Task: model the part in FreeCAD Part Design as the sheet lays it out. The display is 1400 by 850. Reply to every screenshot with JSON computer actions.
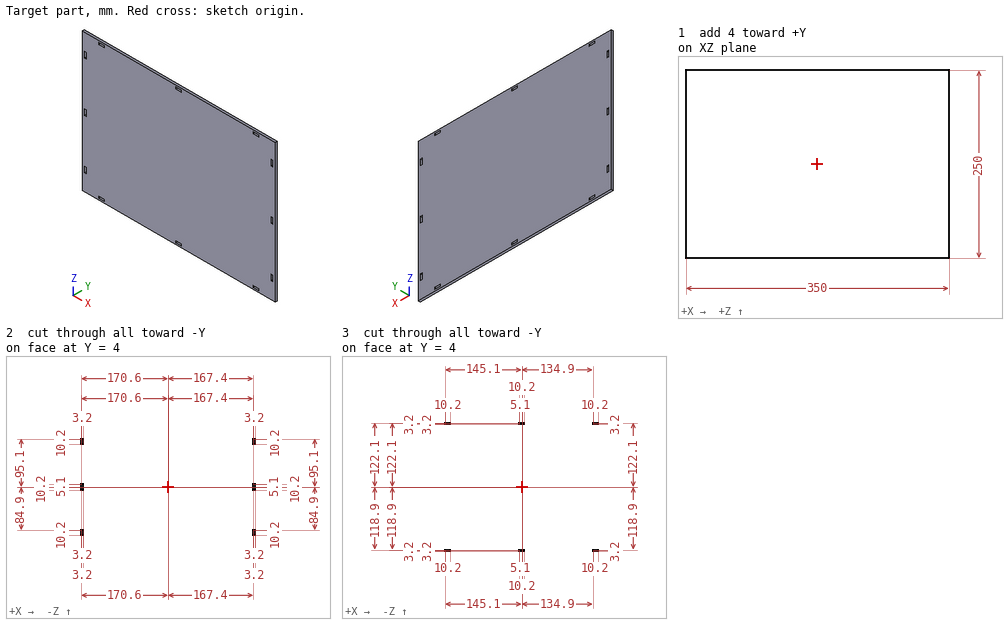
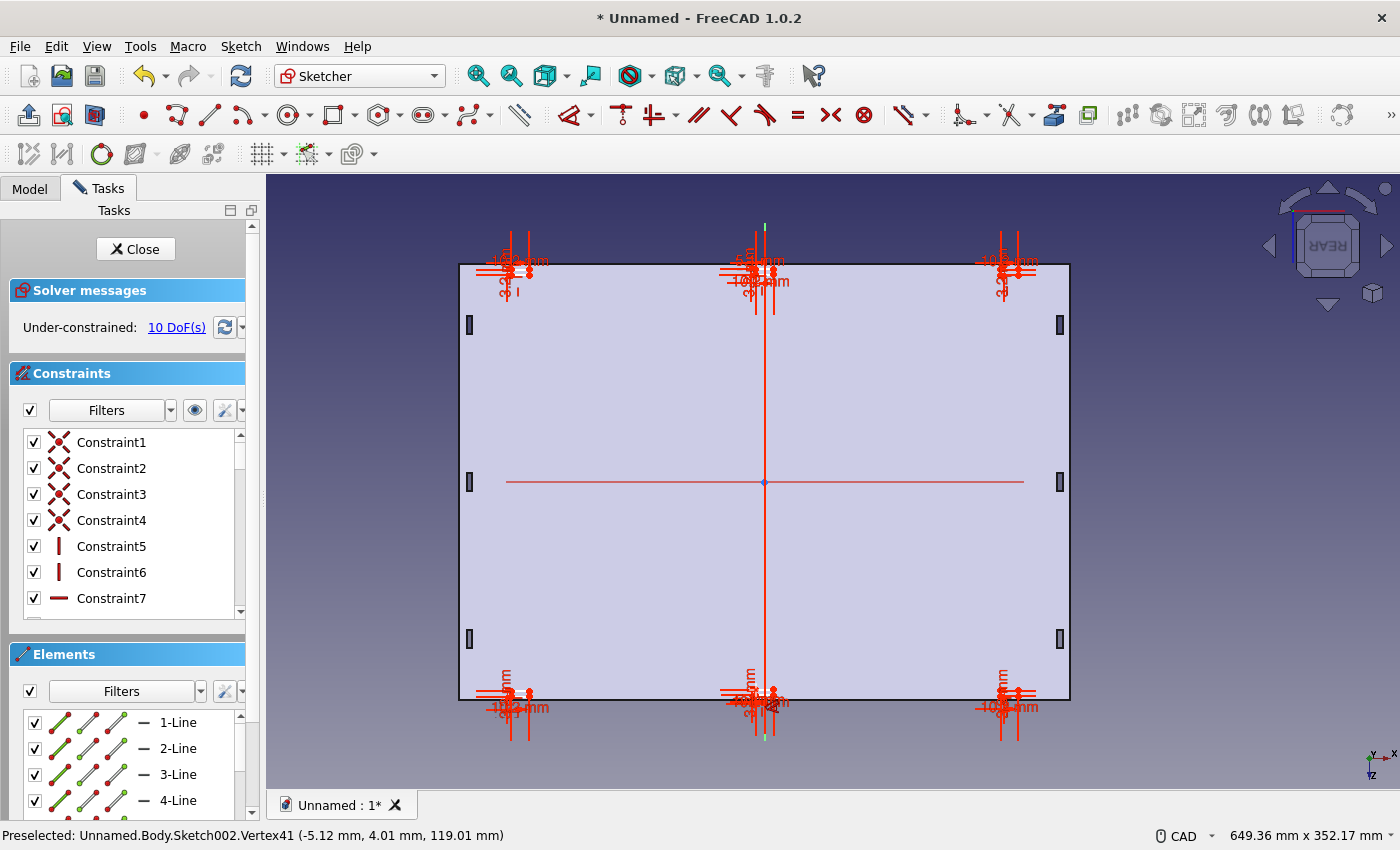
{"action": "scroll", "coordinate": [756, 269], "scroll_direction": "up", "scroll_amount": 4}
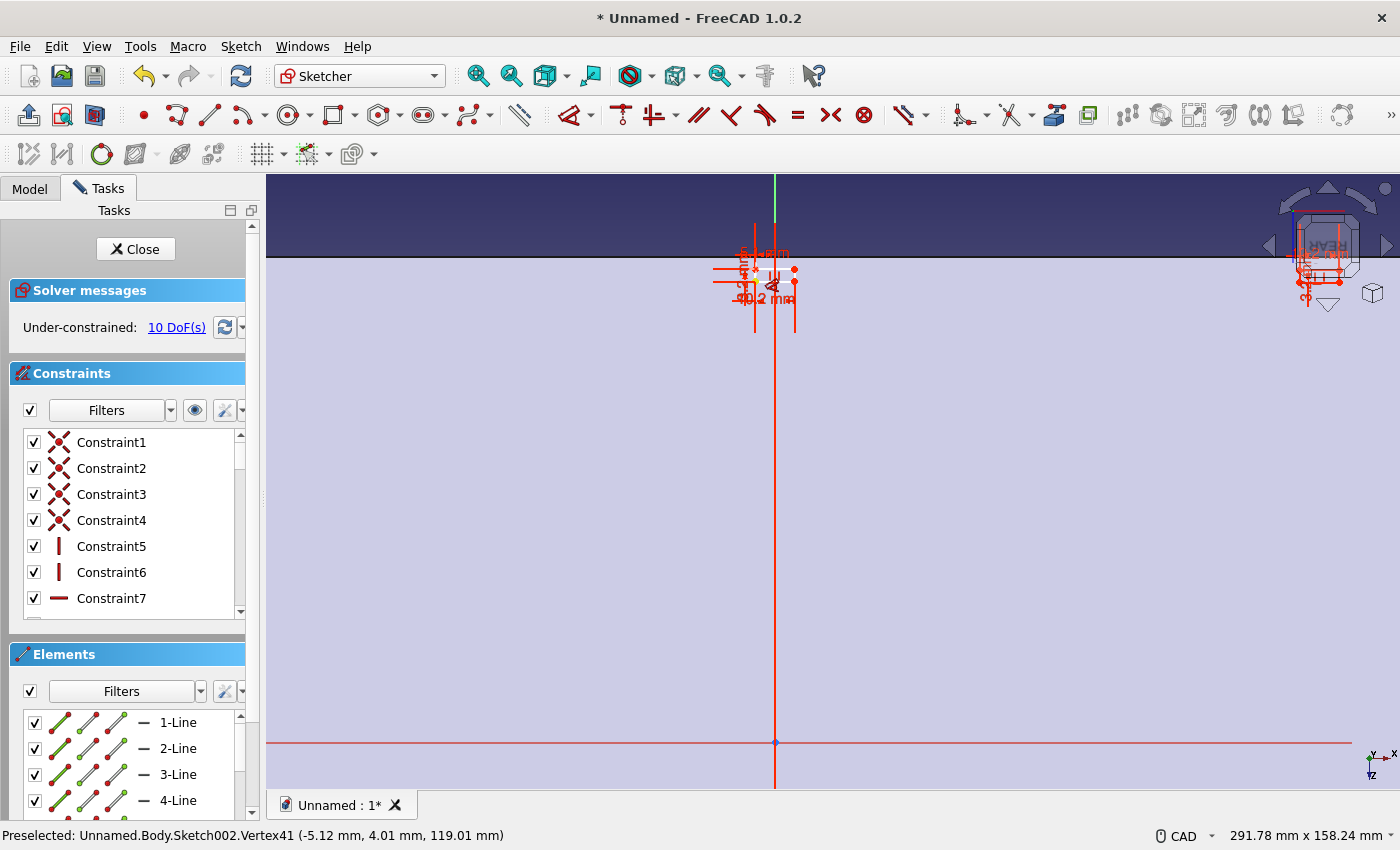
{"action": "left_click", "coordinate": [755, 269]}
{"action": "left_click", "coordinate": [721, 506]}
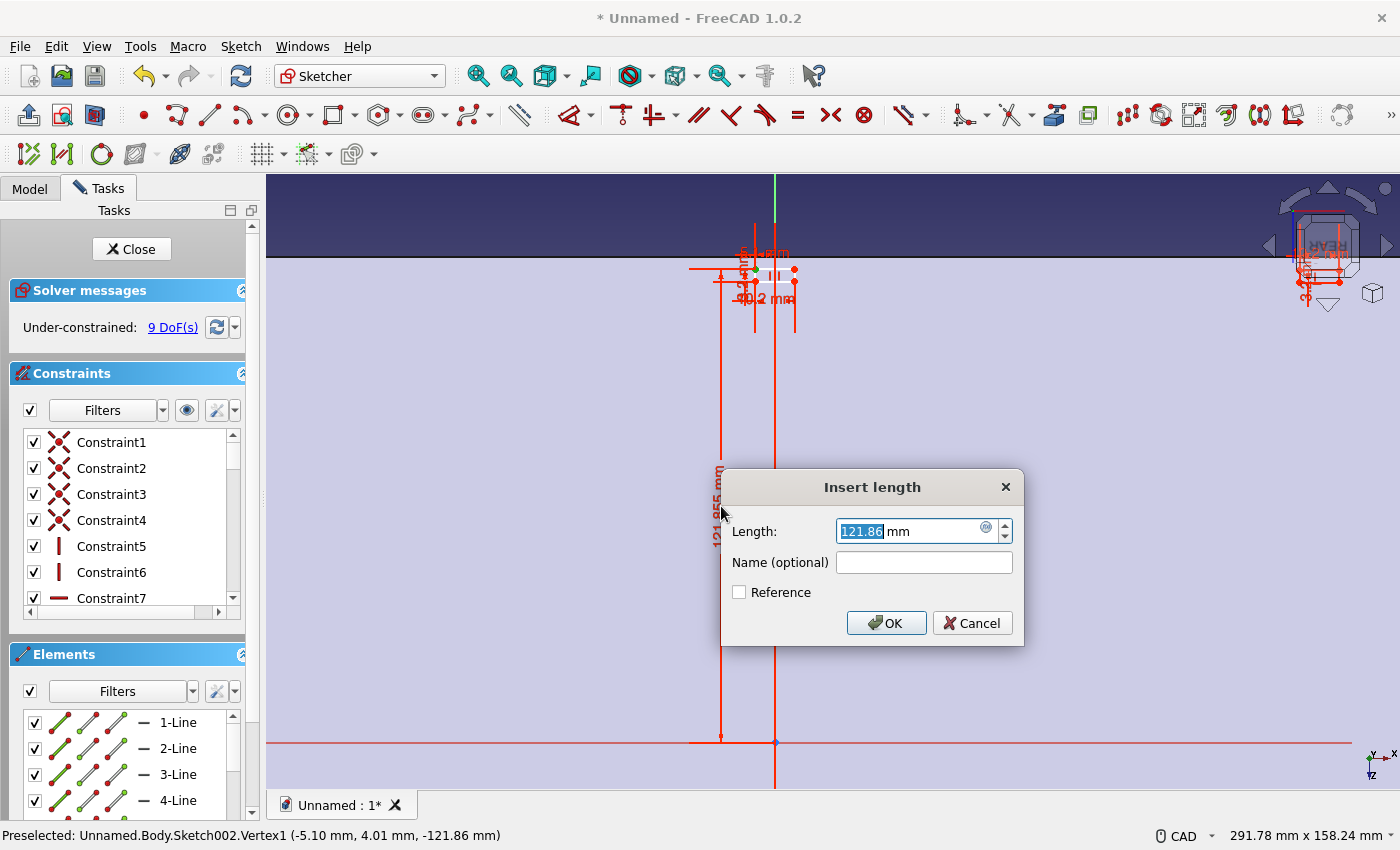
{"action": "type", "text": "122.1"}
{"action": "key", "text": "Return"}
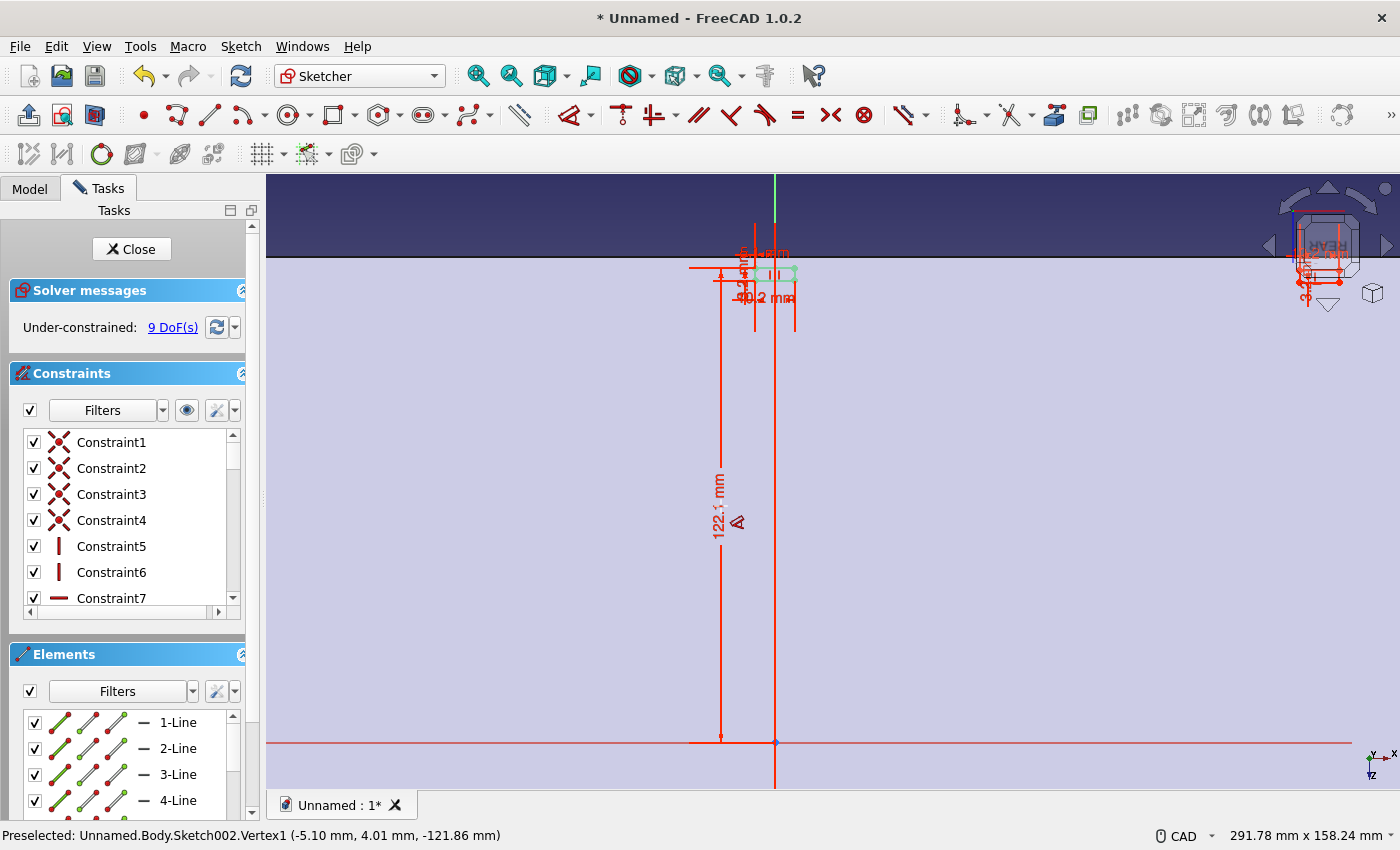
{"action": "scroll", "coordinate": [756, 268], "scroll_direction": "down", "scroll_amount": 4}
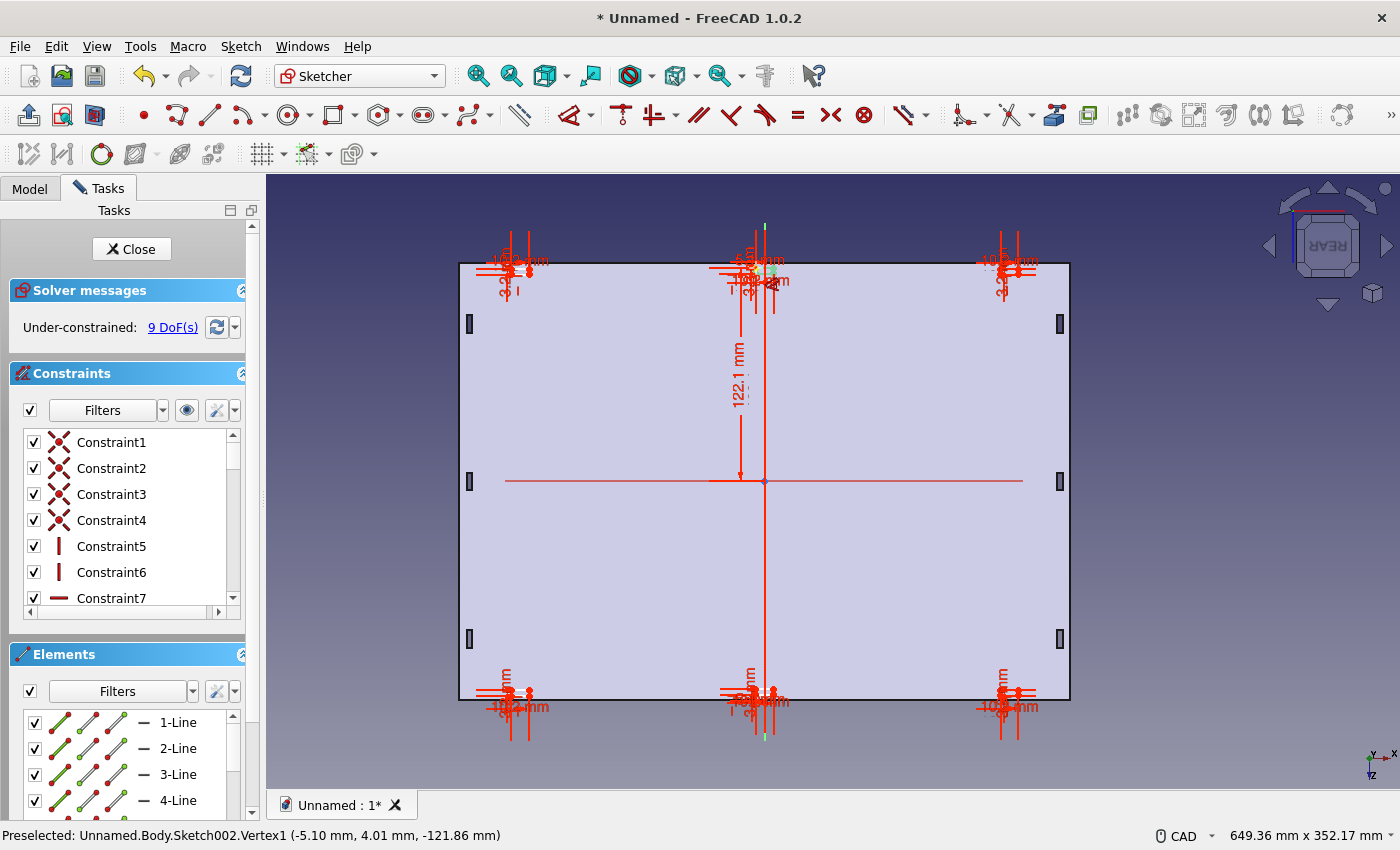
{"action": "scroll", "coordinate": [1001, 269], "scroll_direction": "up", "scroll_amount": 4}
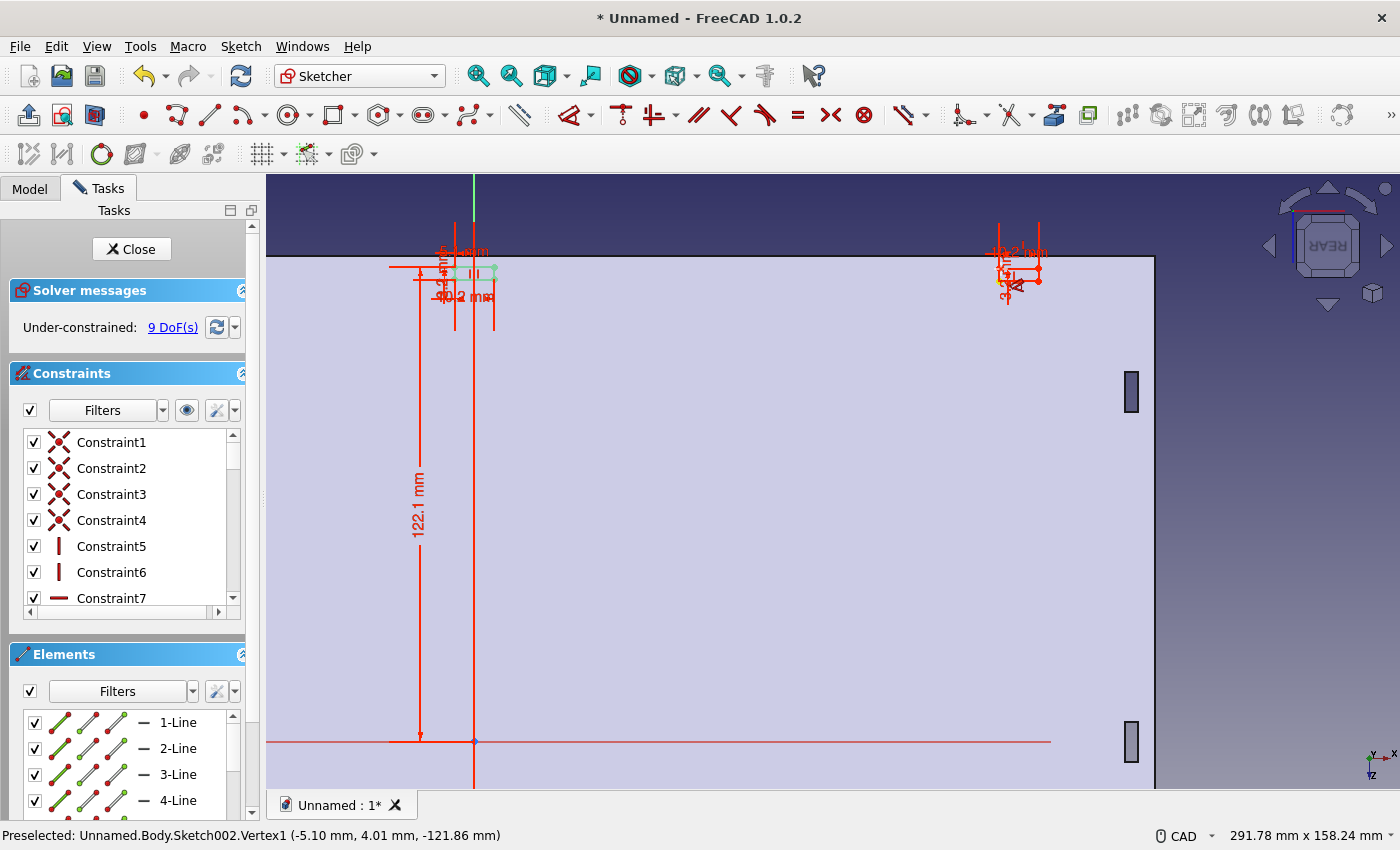
{"action": "left_click", "coordinate": [999, 269]}
{"action": "left_click", "coordinate": [737, 235]}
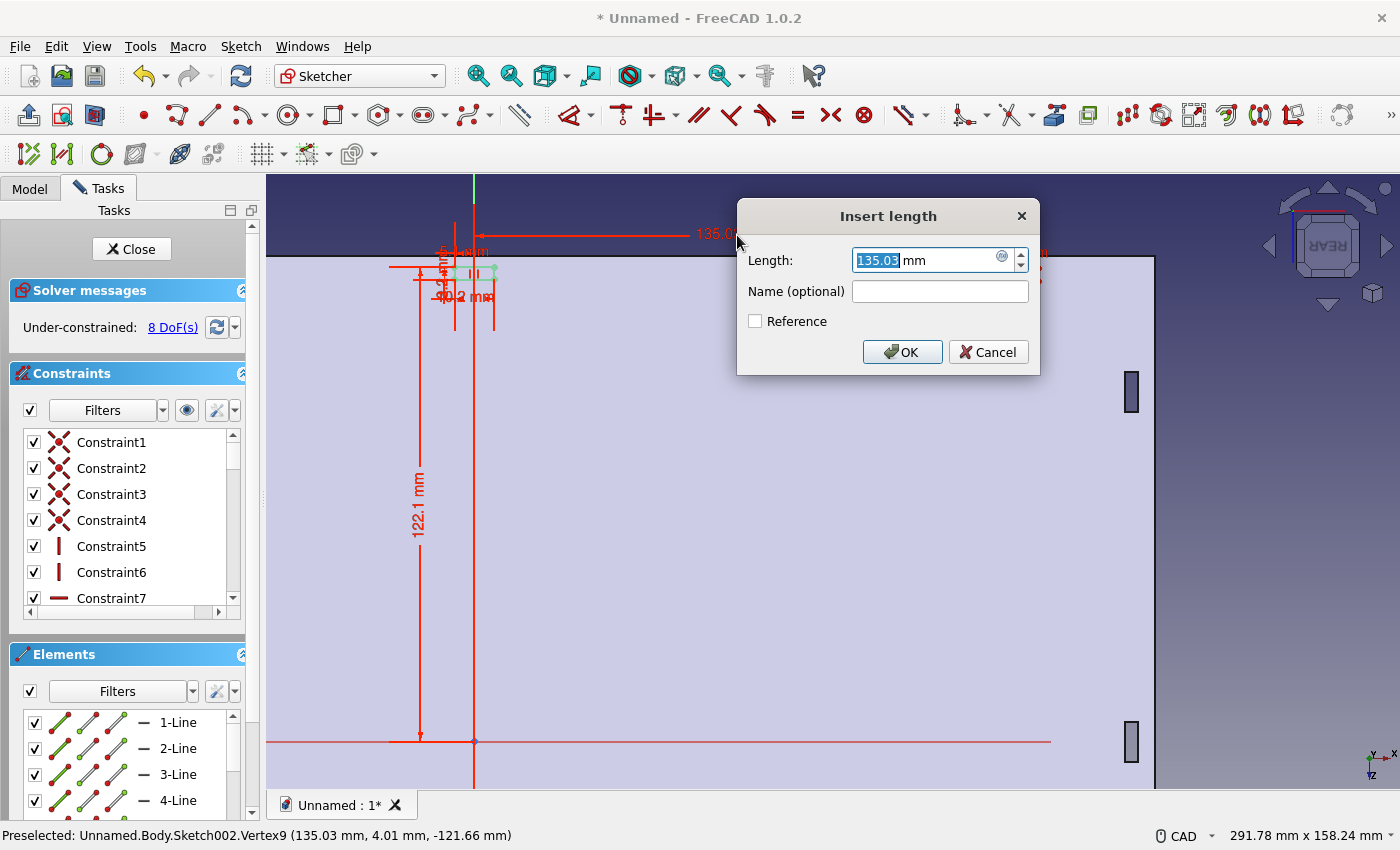
{"action": "type", "text": "134.9"}
{"action": "key", "text": "Return"}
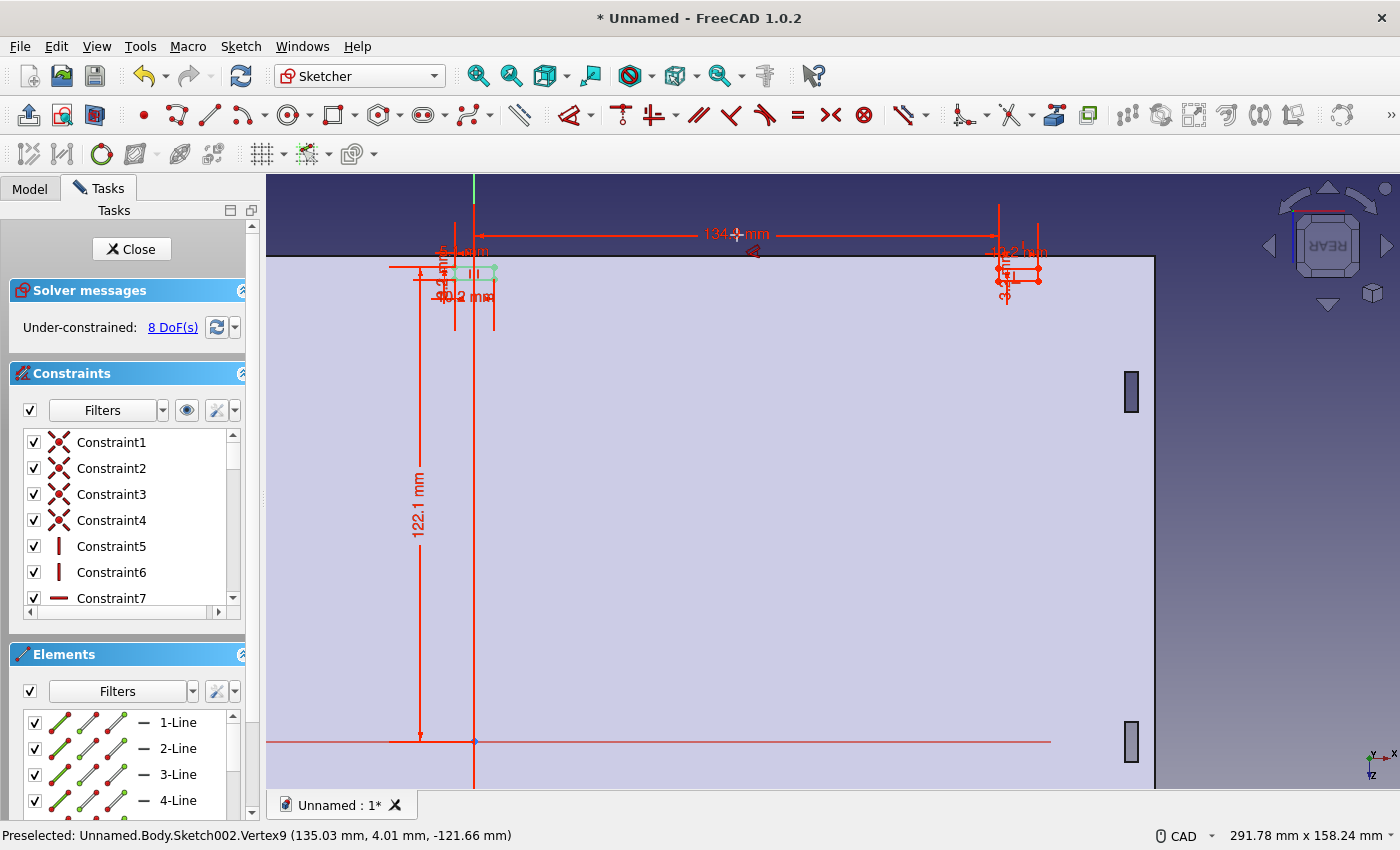
{"action": "left_click", "coordinate": [999, 269]}
{"action": "left_click", "coordinate": [1033, 505]}